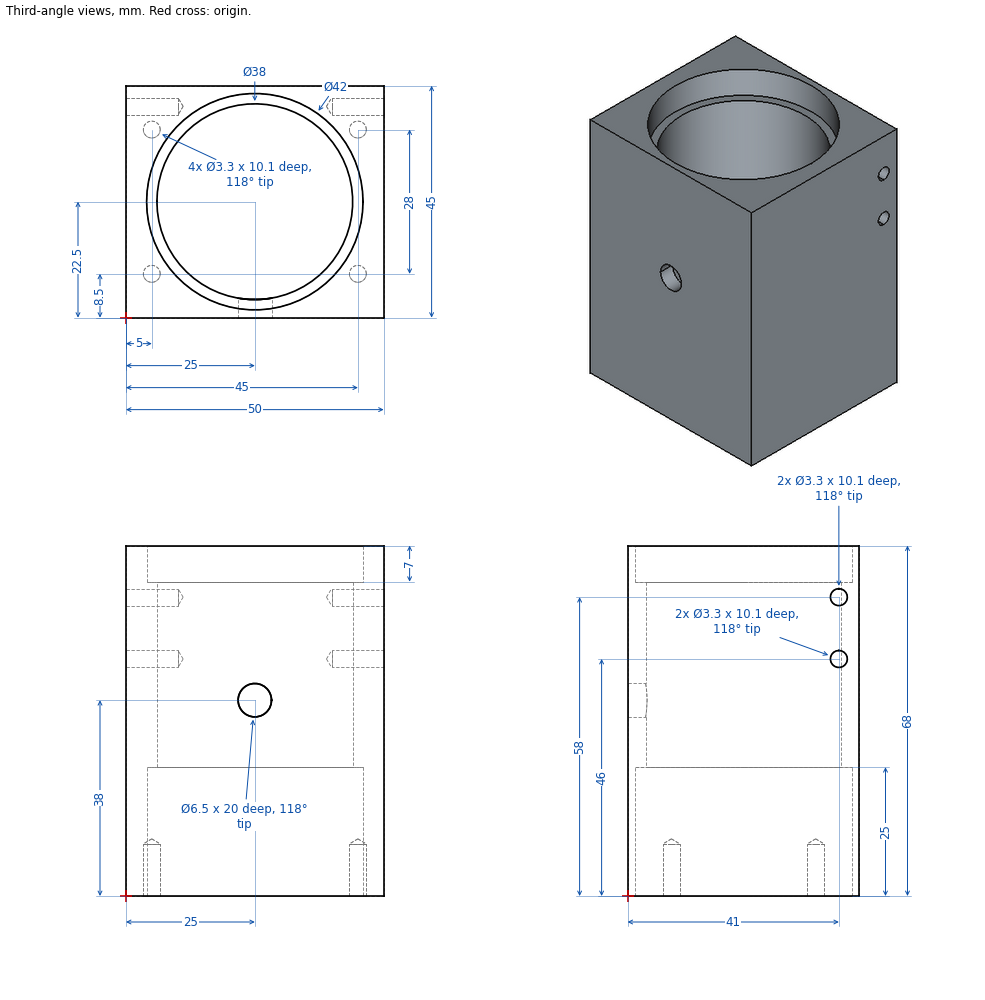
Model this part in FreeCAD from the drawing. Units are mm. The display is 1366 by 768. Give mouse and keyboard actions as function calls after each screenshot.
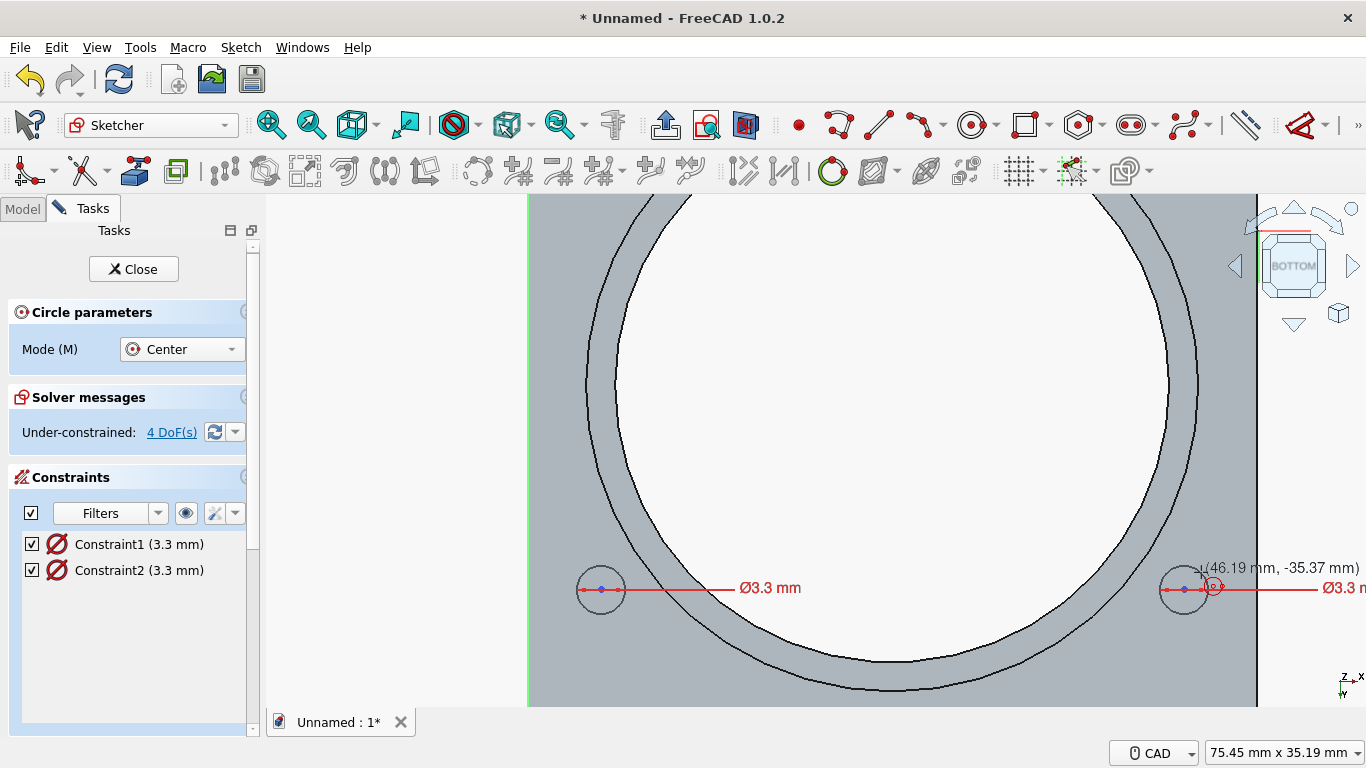
scroll(601, 591, down, 3)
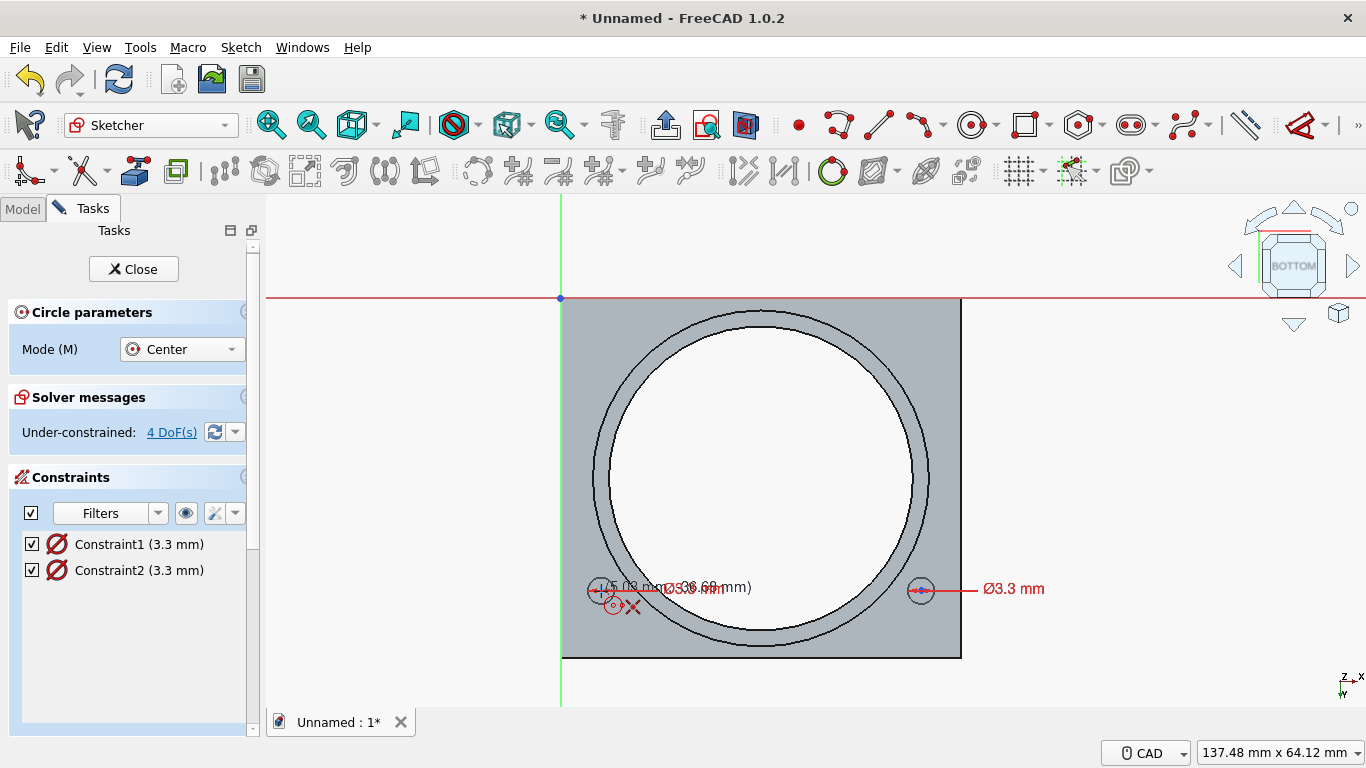
scroll(921, 366, up, 3)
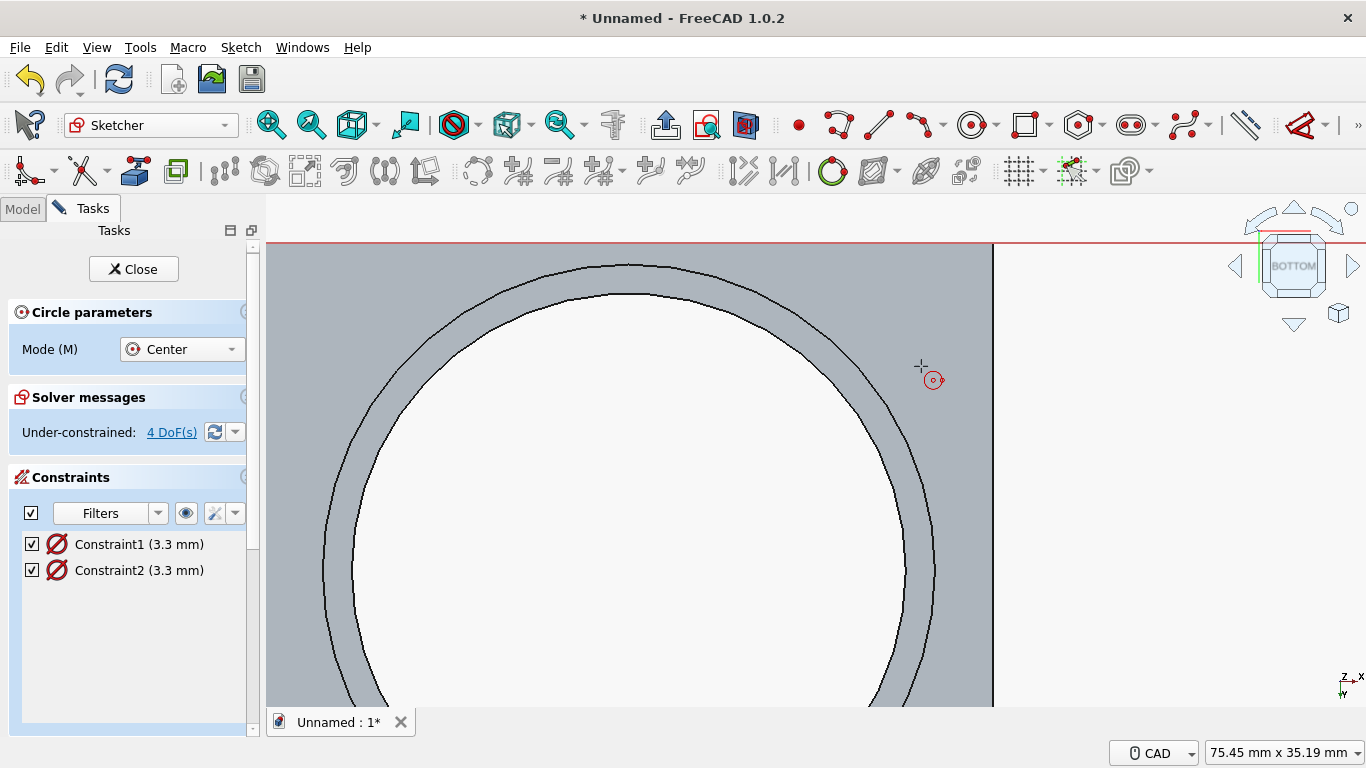
click(920, 367)
move(937, 350)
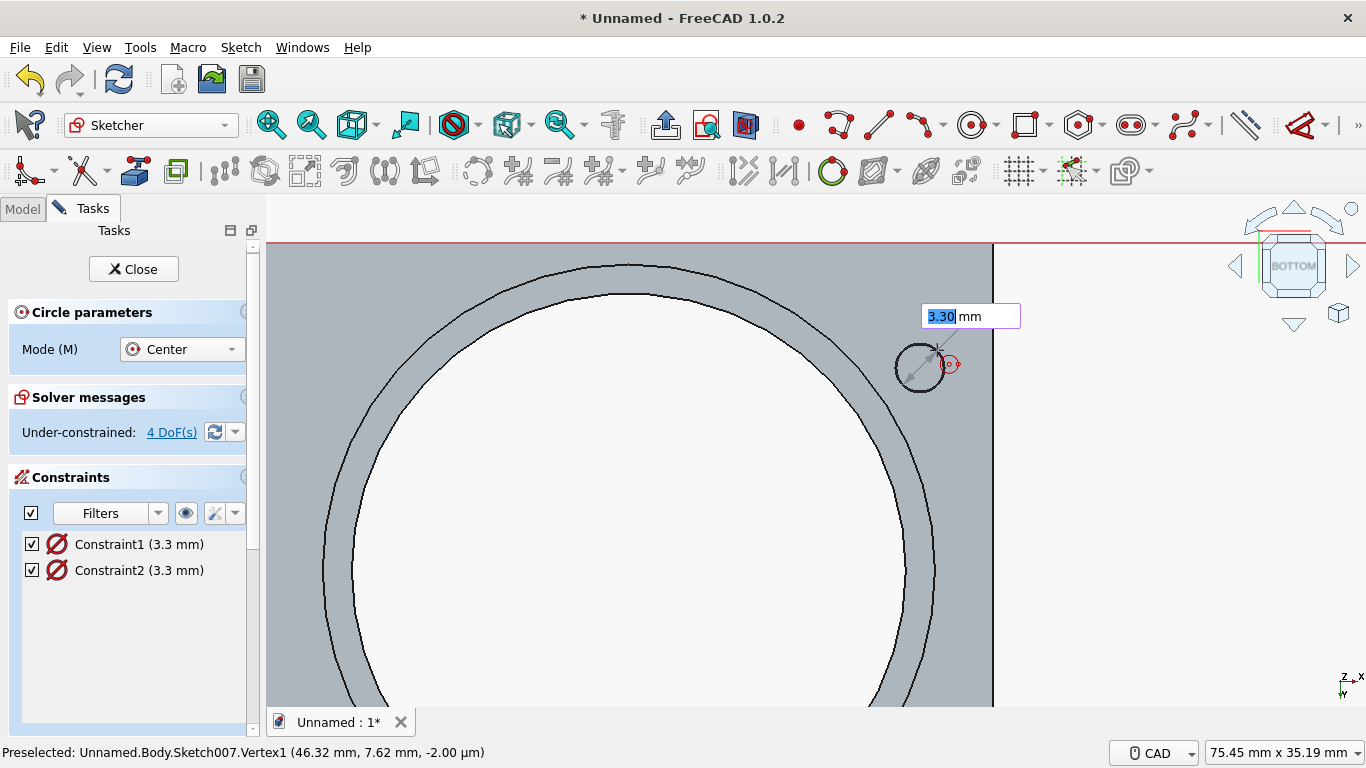
text(3.3)
key(Return)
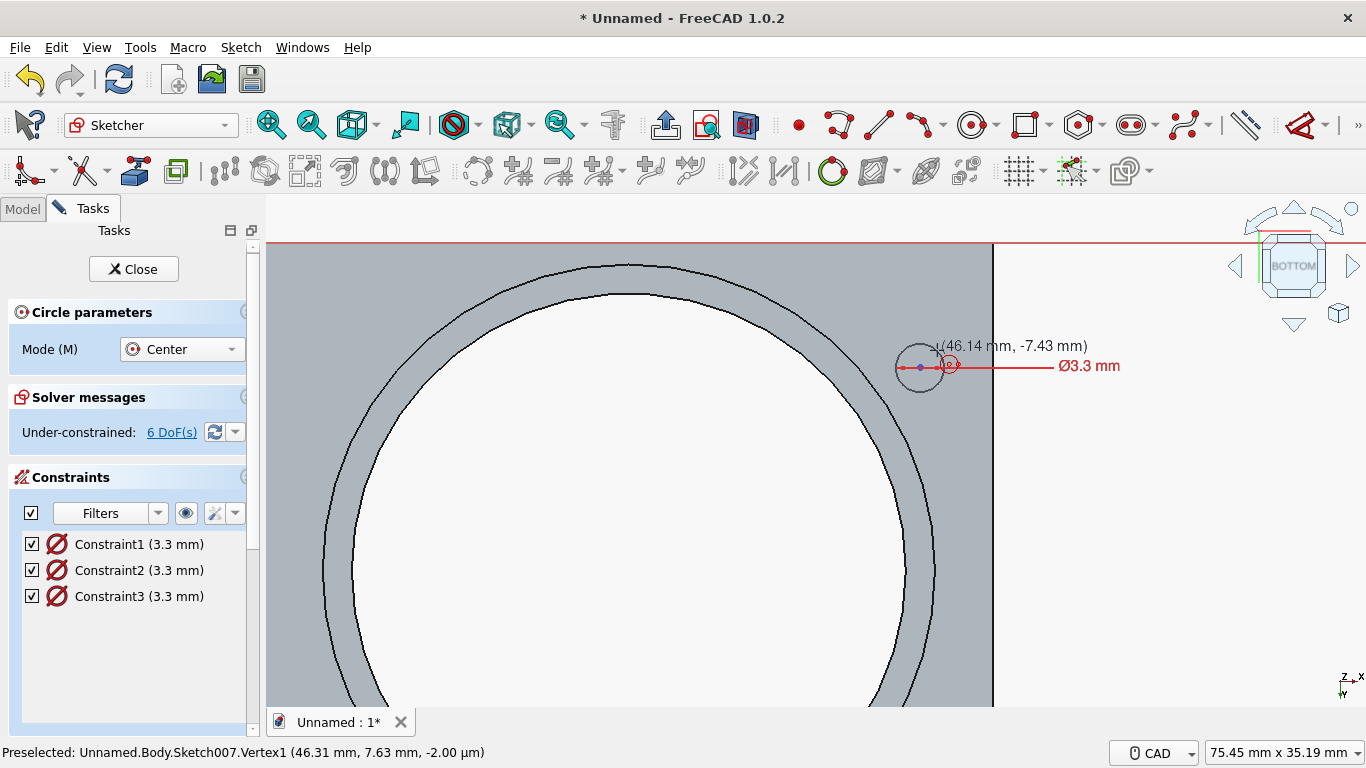
click(337, 367)
move(354, 350)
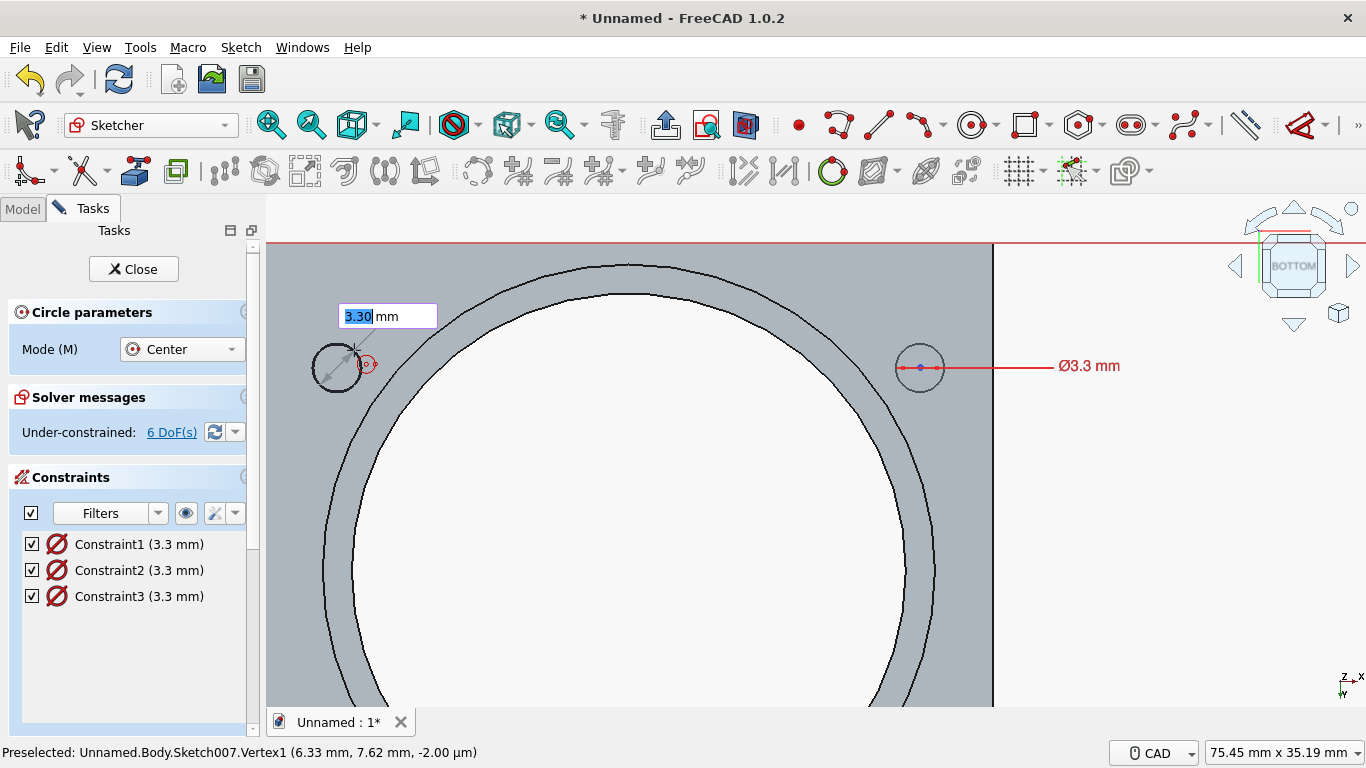
text(3.3)
key(Return)
key(Escape)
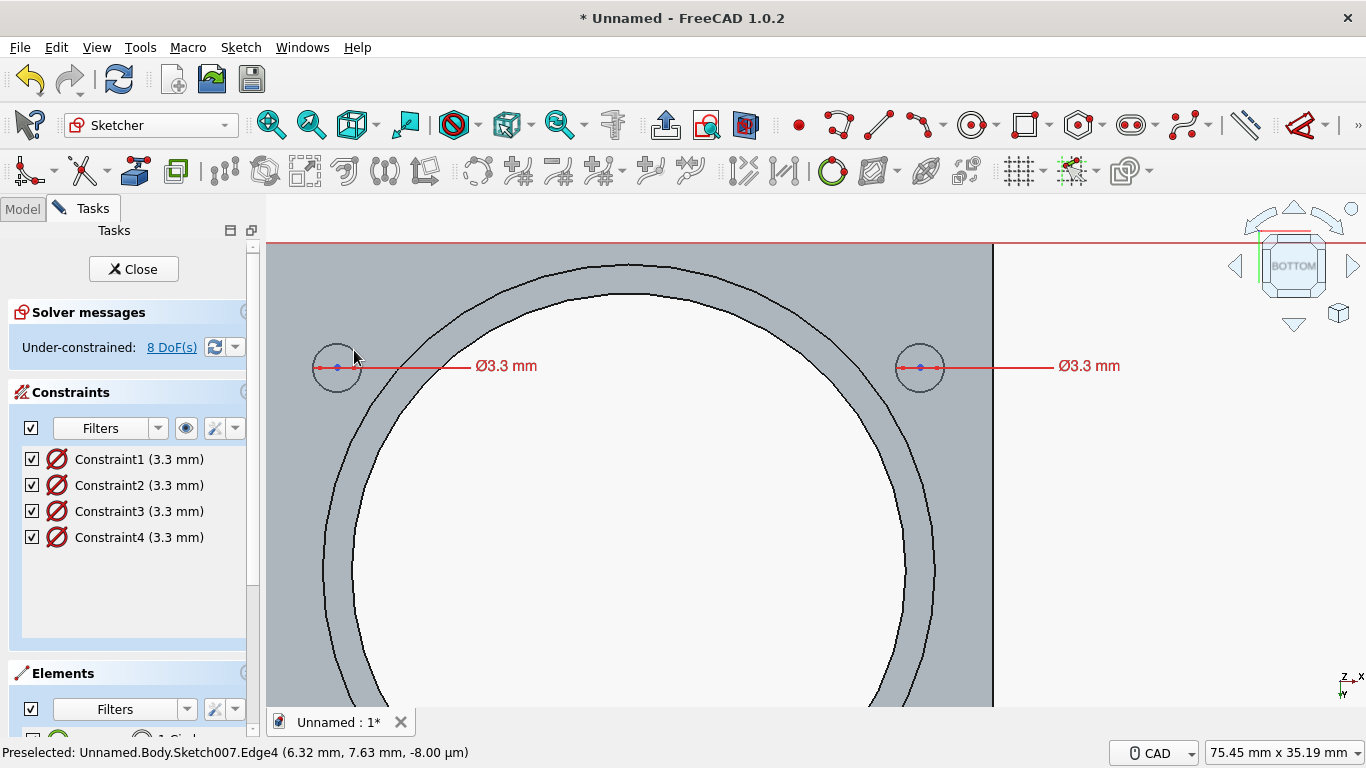
scroll(922, 365, down, 3)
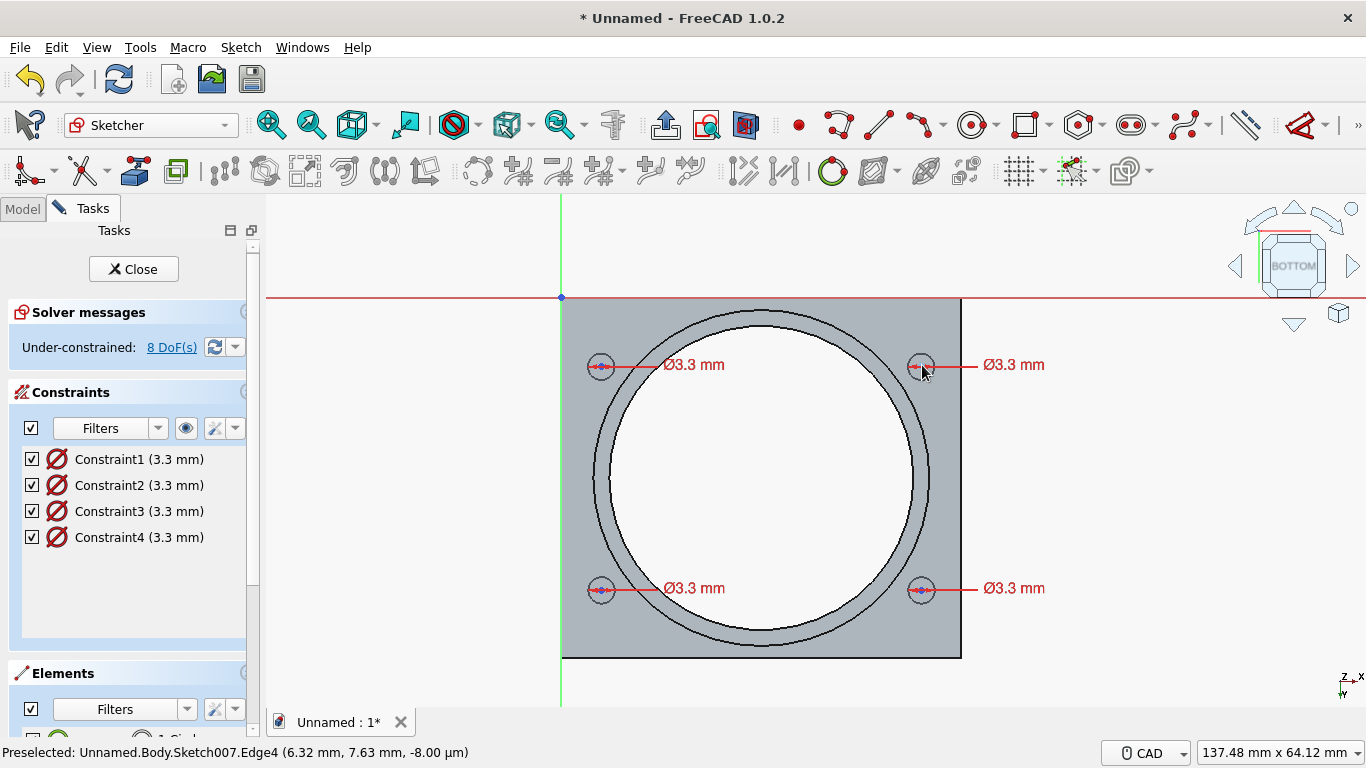
click(602, 590)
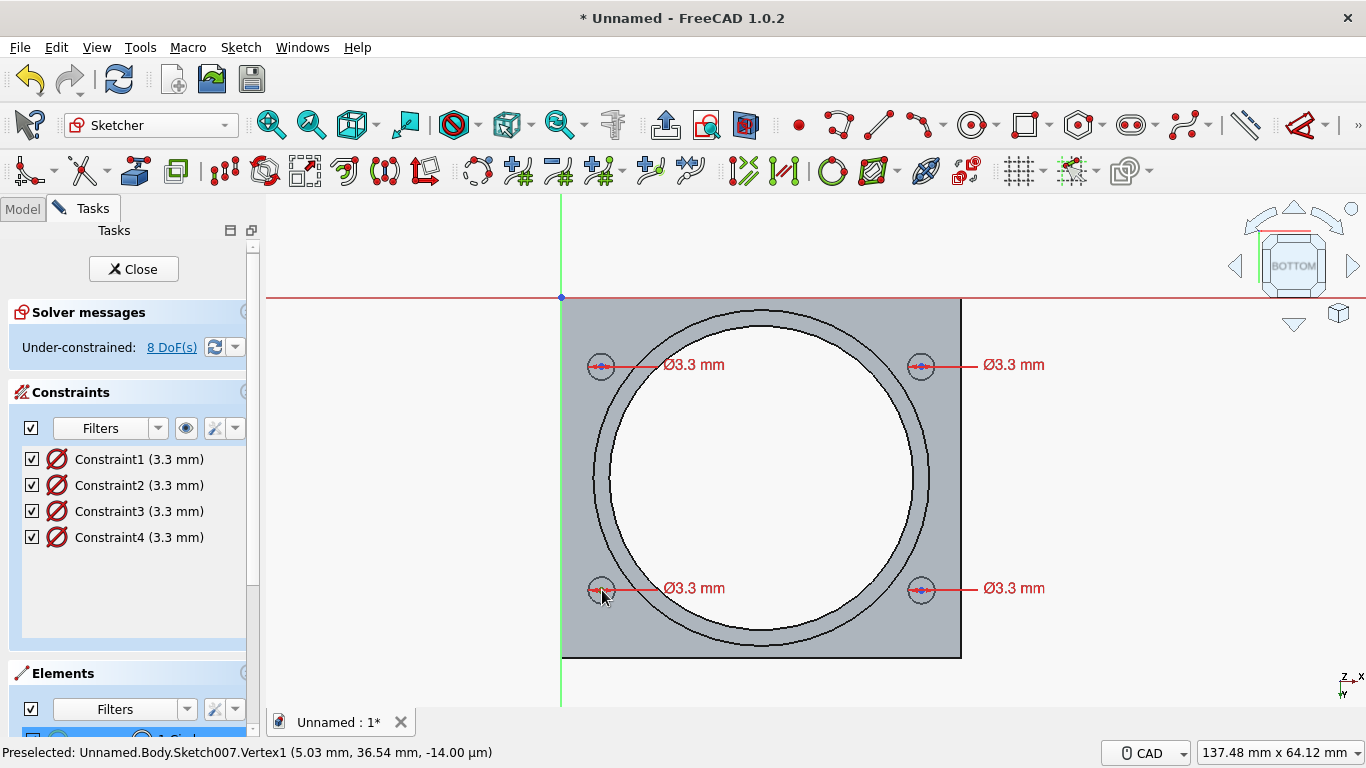
click(922, 590)